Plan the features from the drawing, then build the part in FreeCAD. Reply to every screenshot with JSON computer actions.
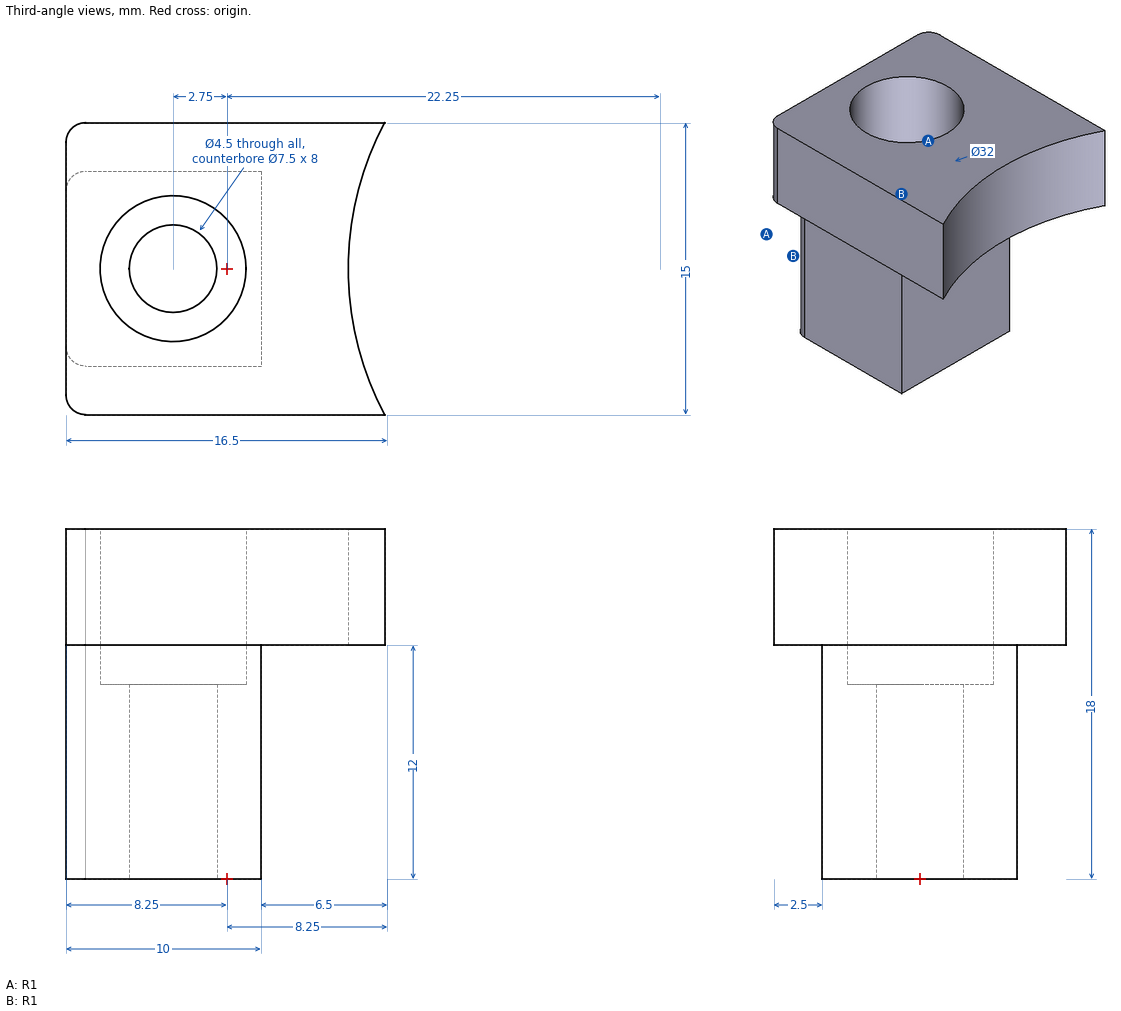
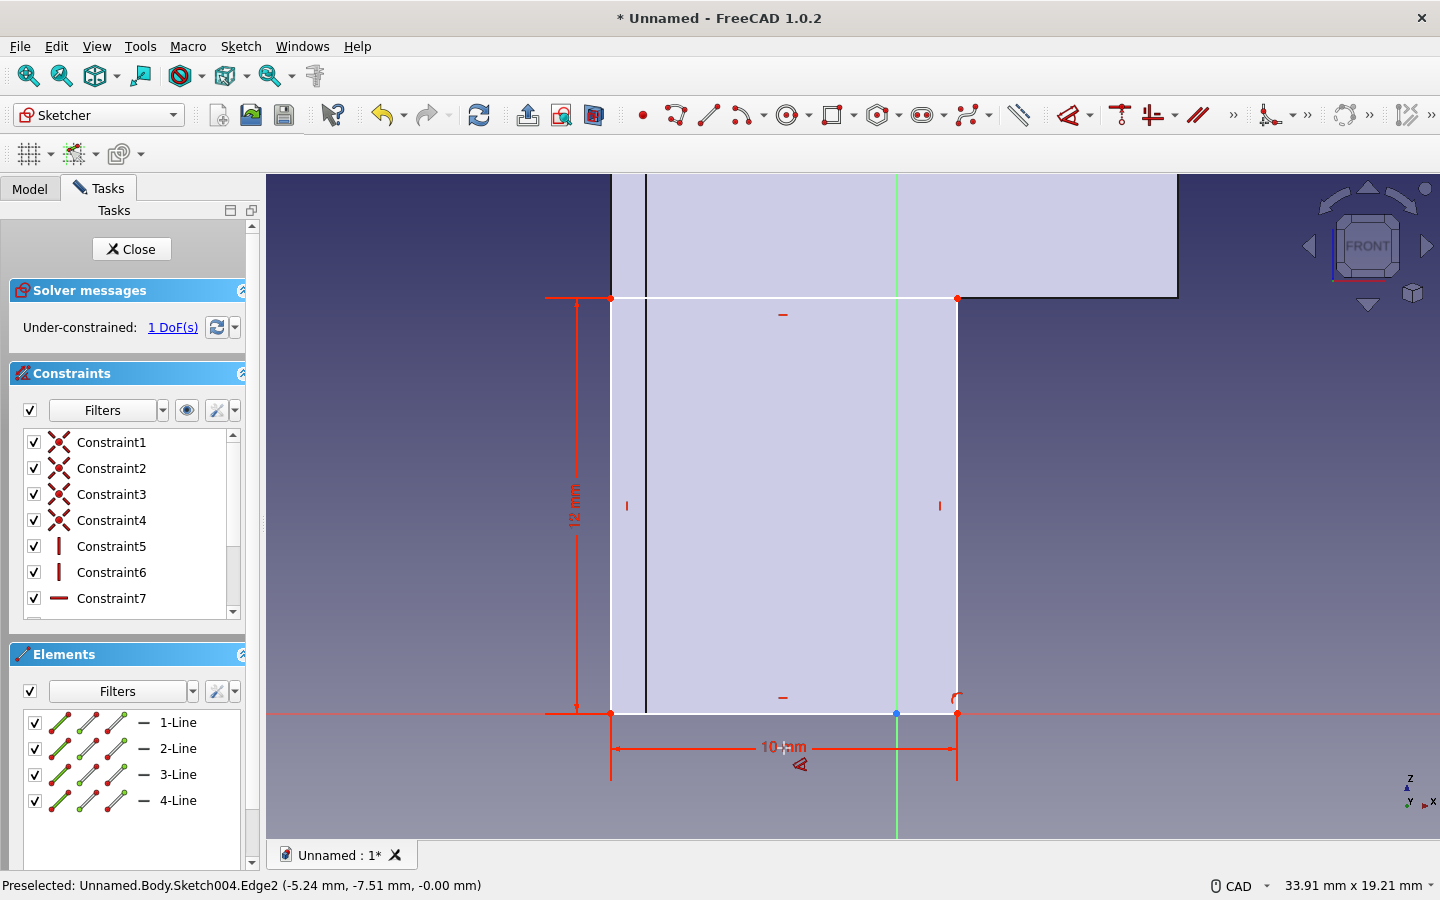
{"action": "left_click", "coordinate": [611, 298]}
{"action": "left_click", "coordinate": [688, 748]}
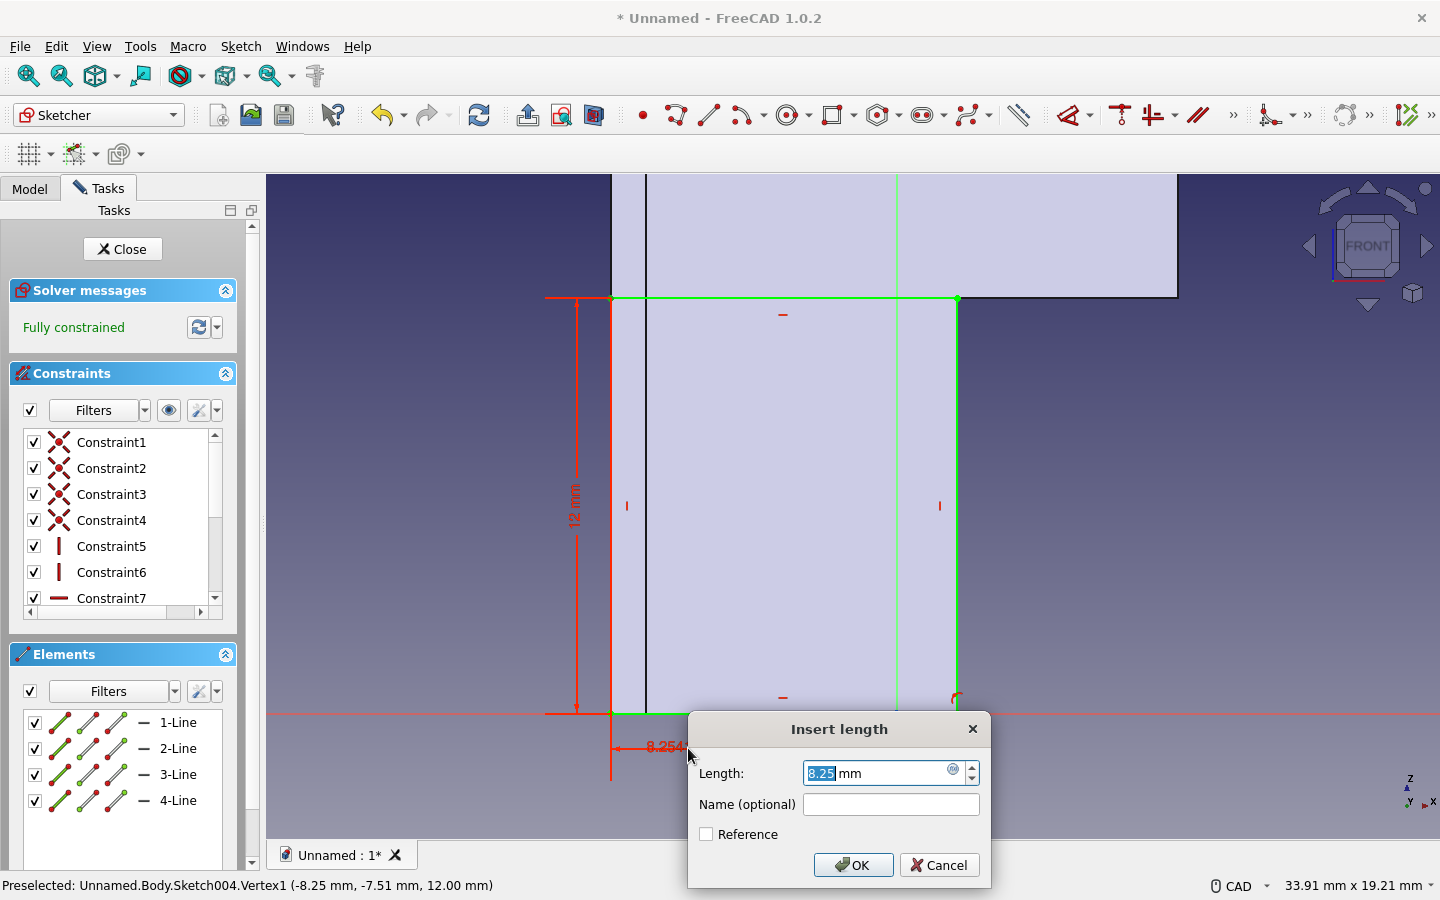
{"action": "type", "text": "8.25"}
{"action": "key", "text": "Return"}
{"action": "key", "text": "Escape"}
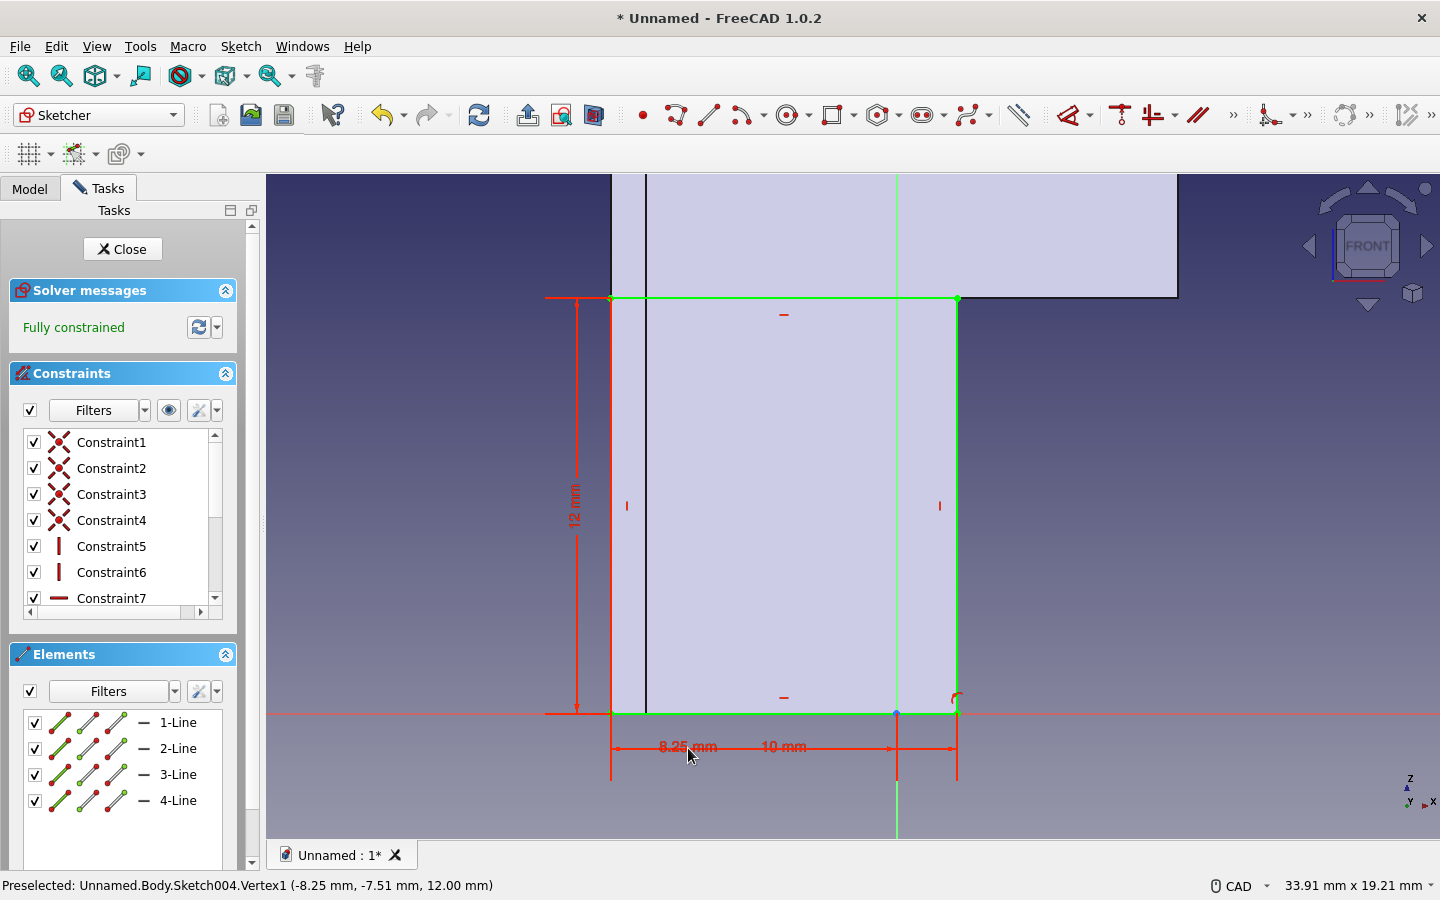
{"action": "left_click", "coordinate": [123, 249]}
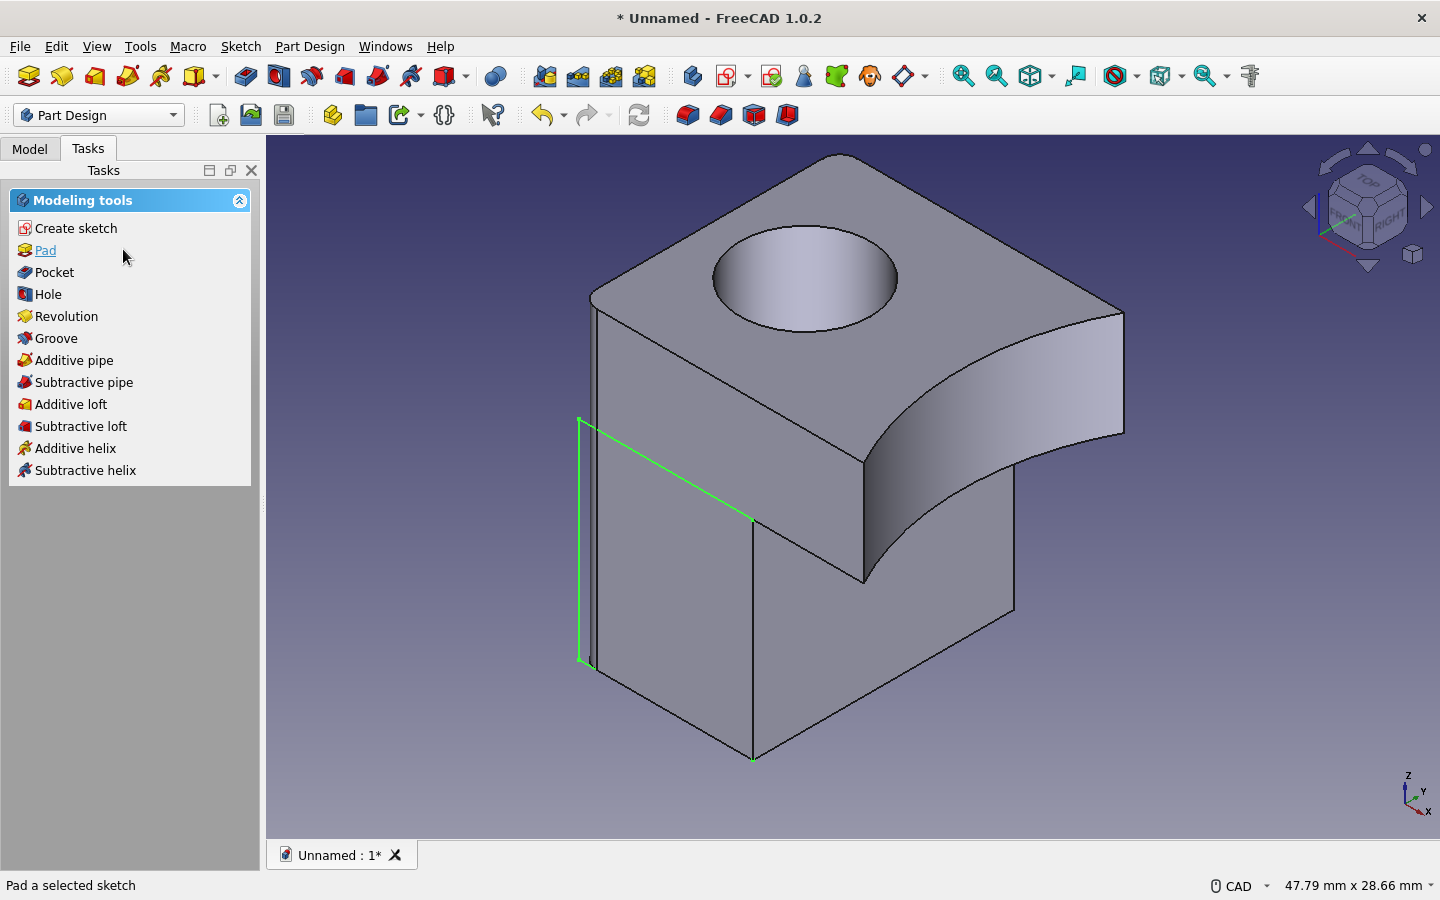
{"action": "left_click", "coordinate": [246, 76]}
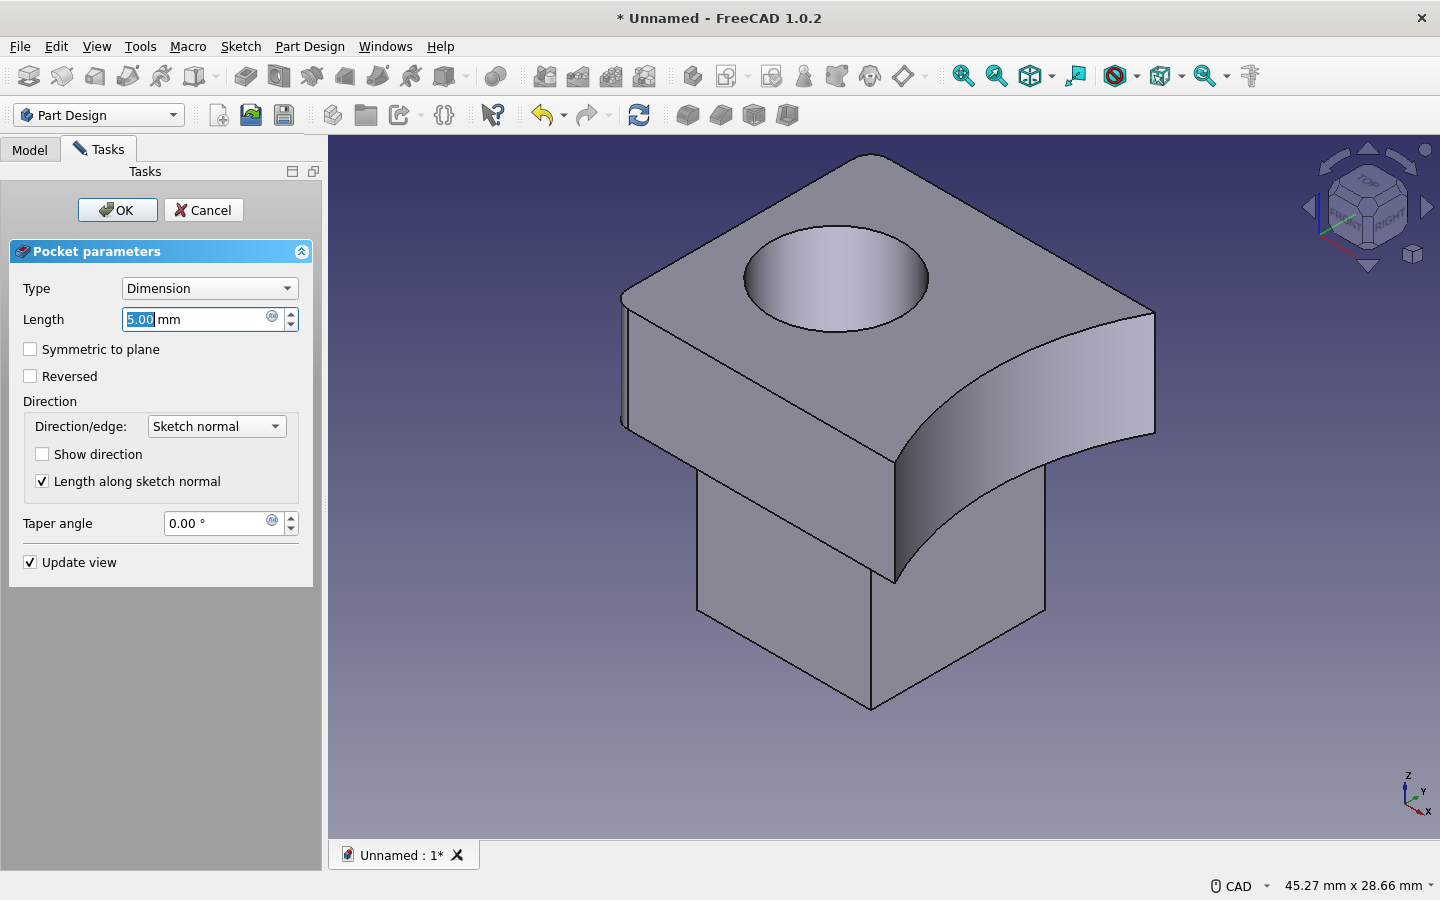
{"action": "type", "text": "2.5"}
{"action": "key", "text": "Tab"}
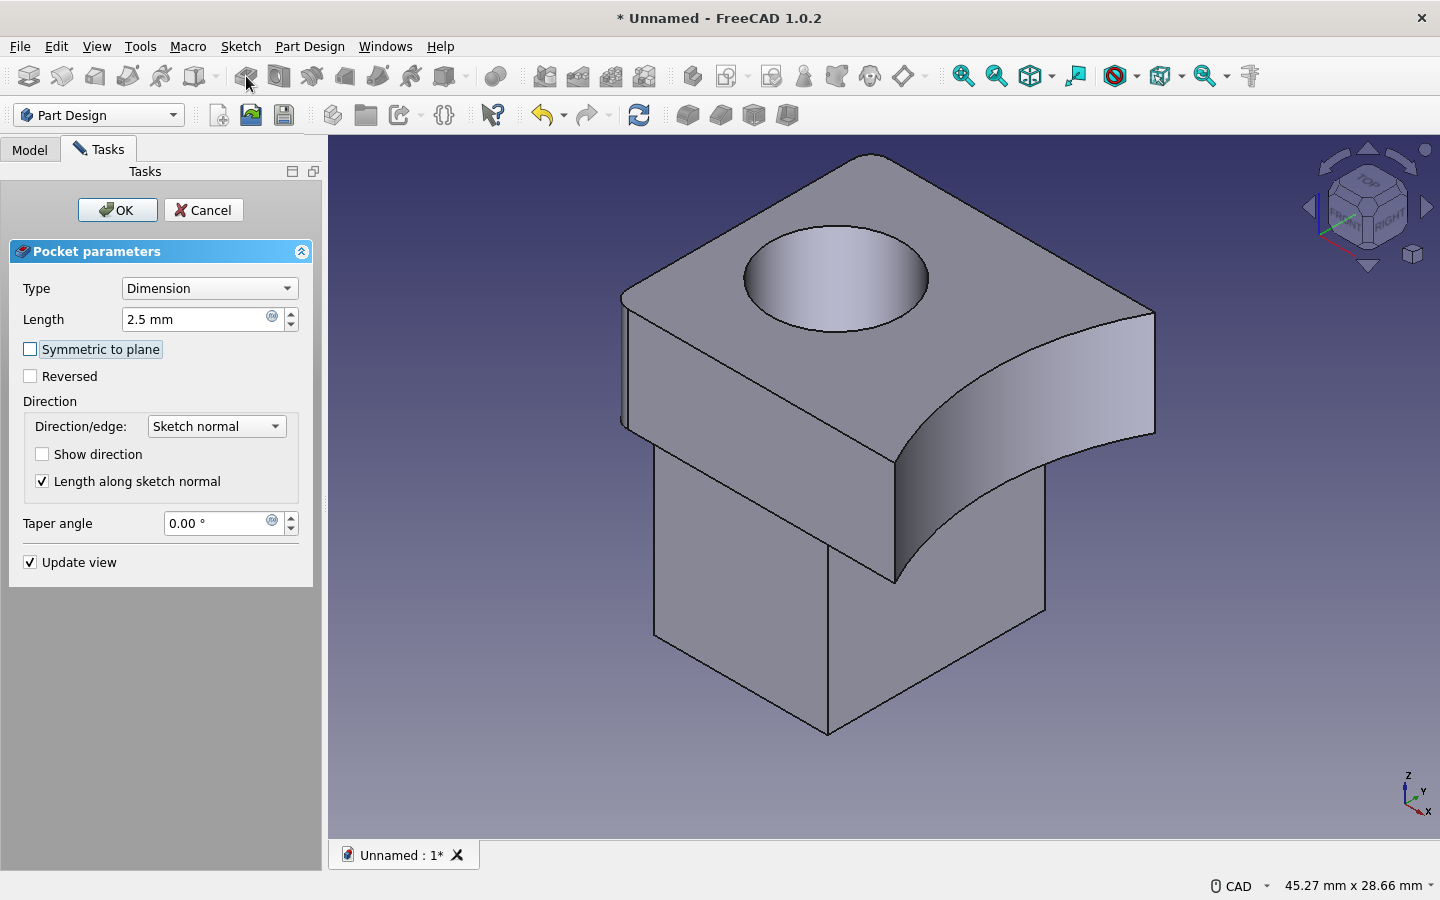
{"action": "left_click", "coordinate": [118, 210]}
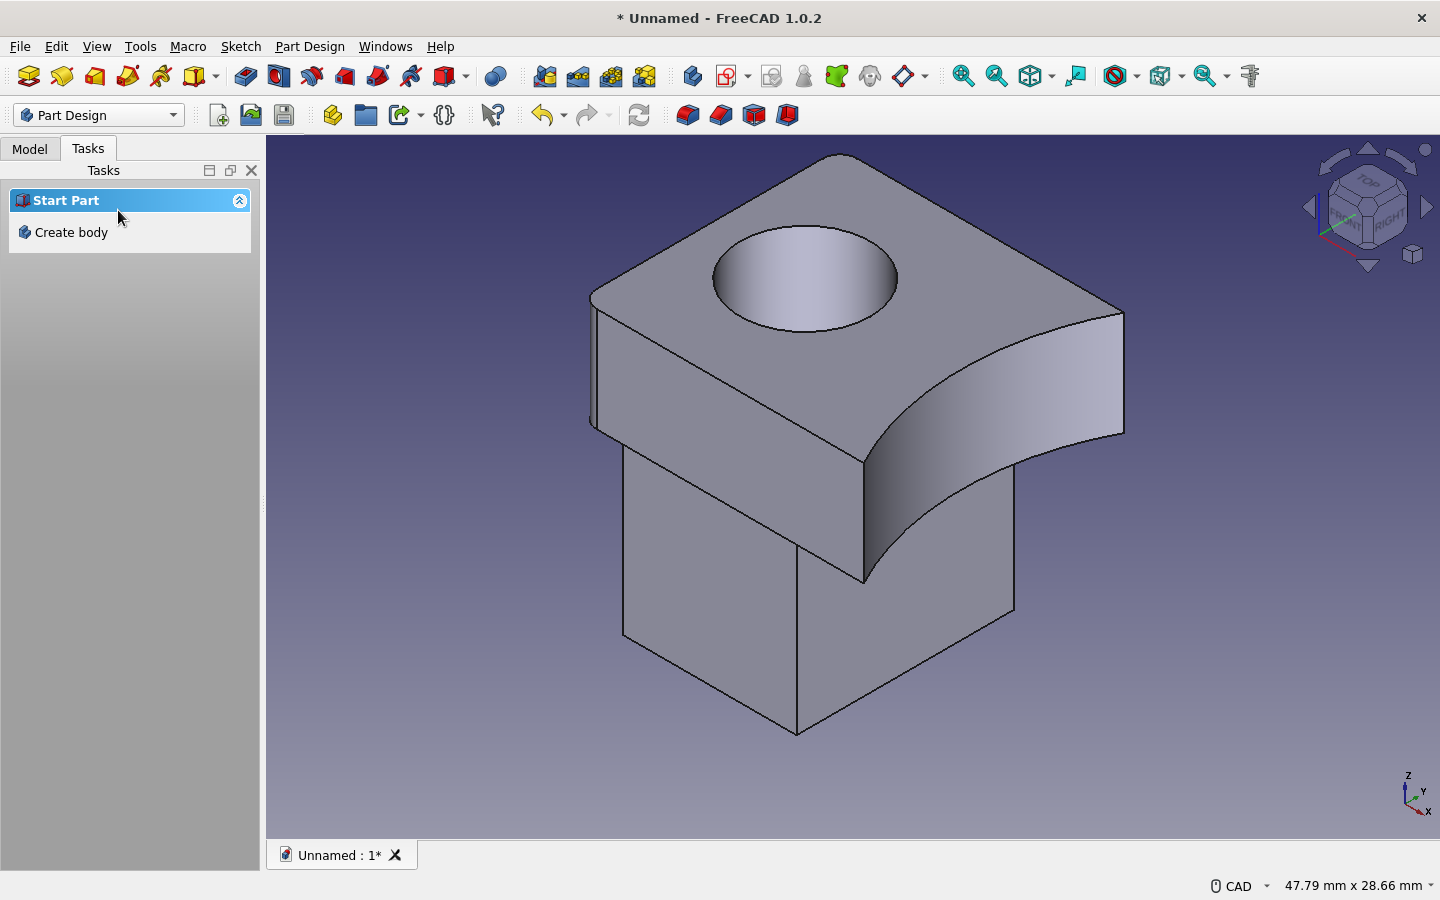
{"action": "left_click", "coordinate": [30, 148]}